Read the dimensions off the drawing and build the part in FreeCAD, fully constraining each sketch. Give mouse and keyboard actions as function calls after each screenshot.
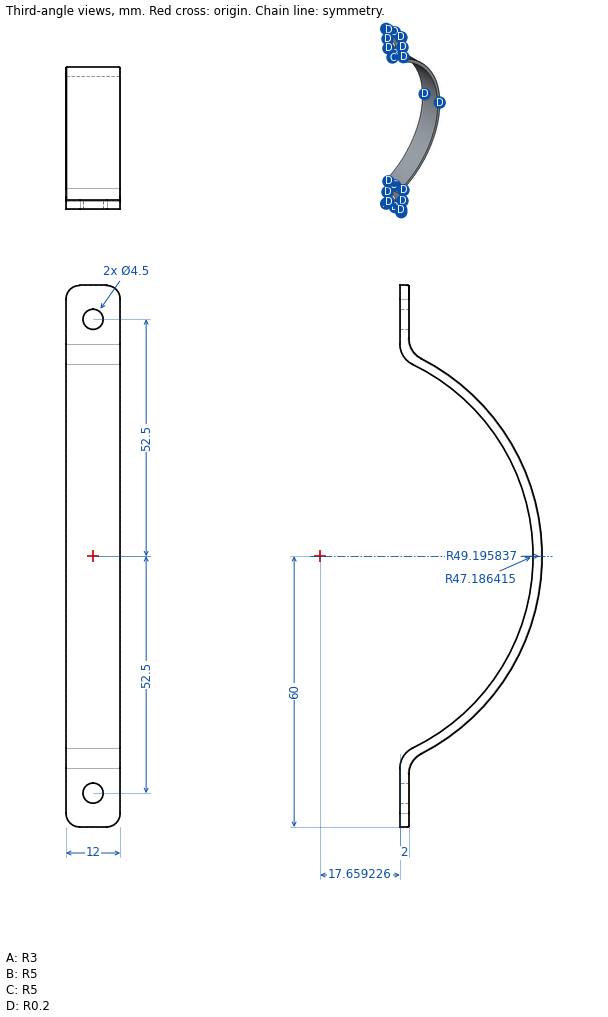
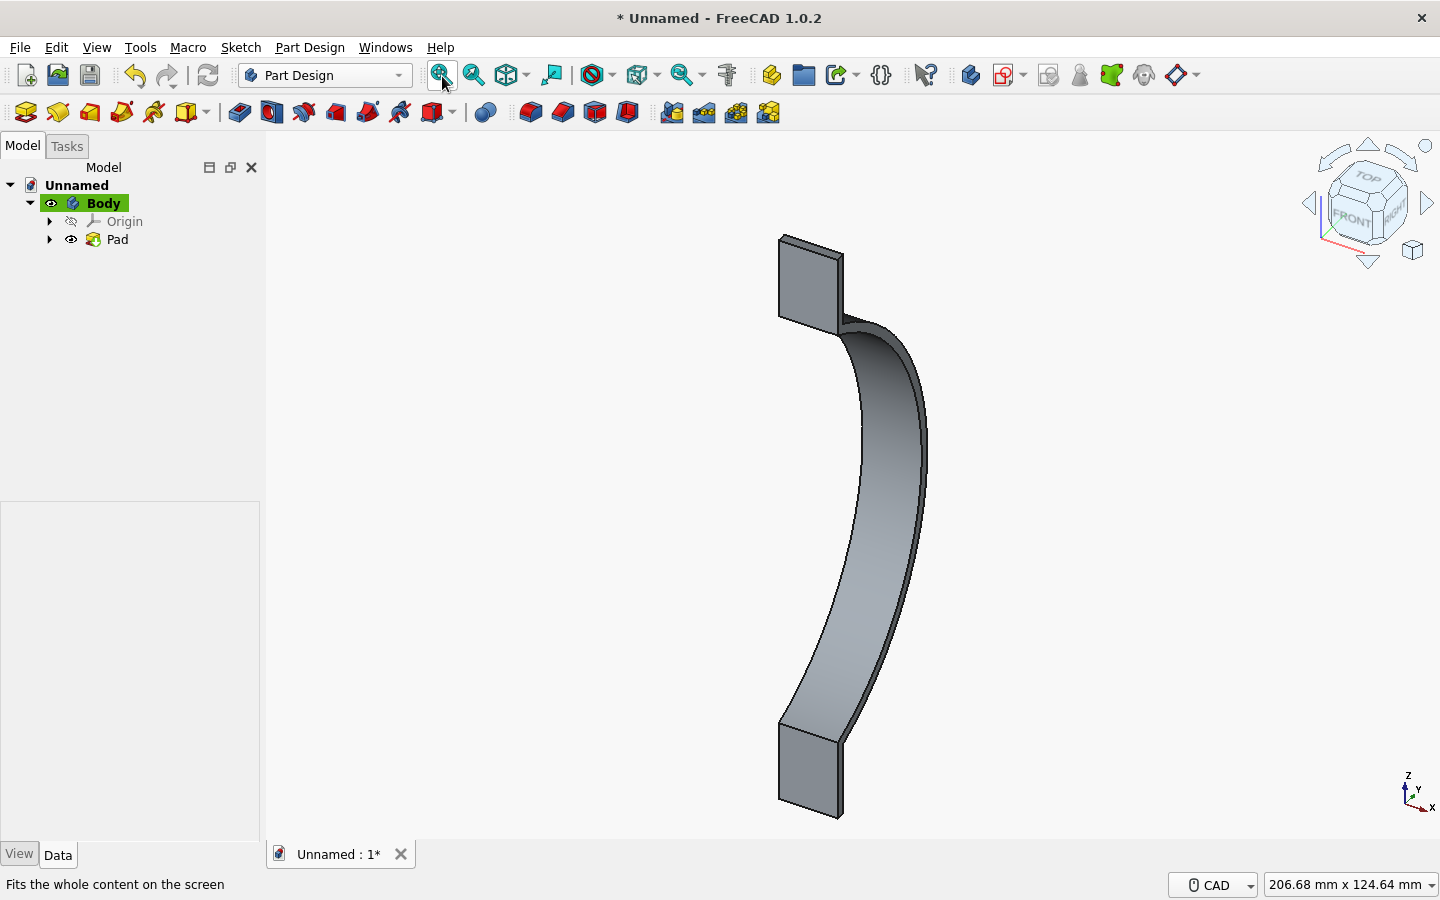
key(4)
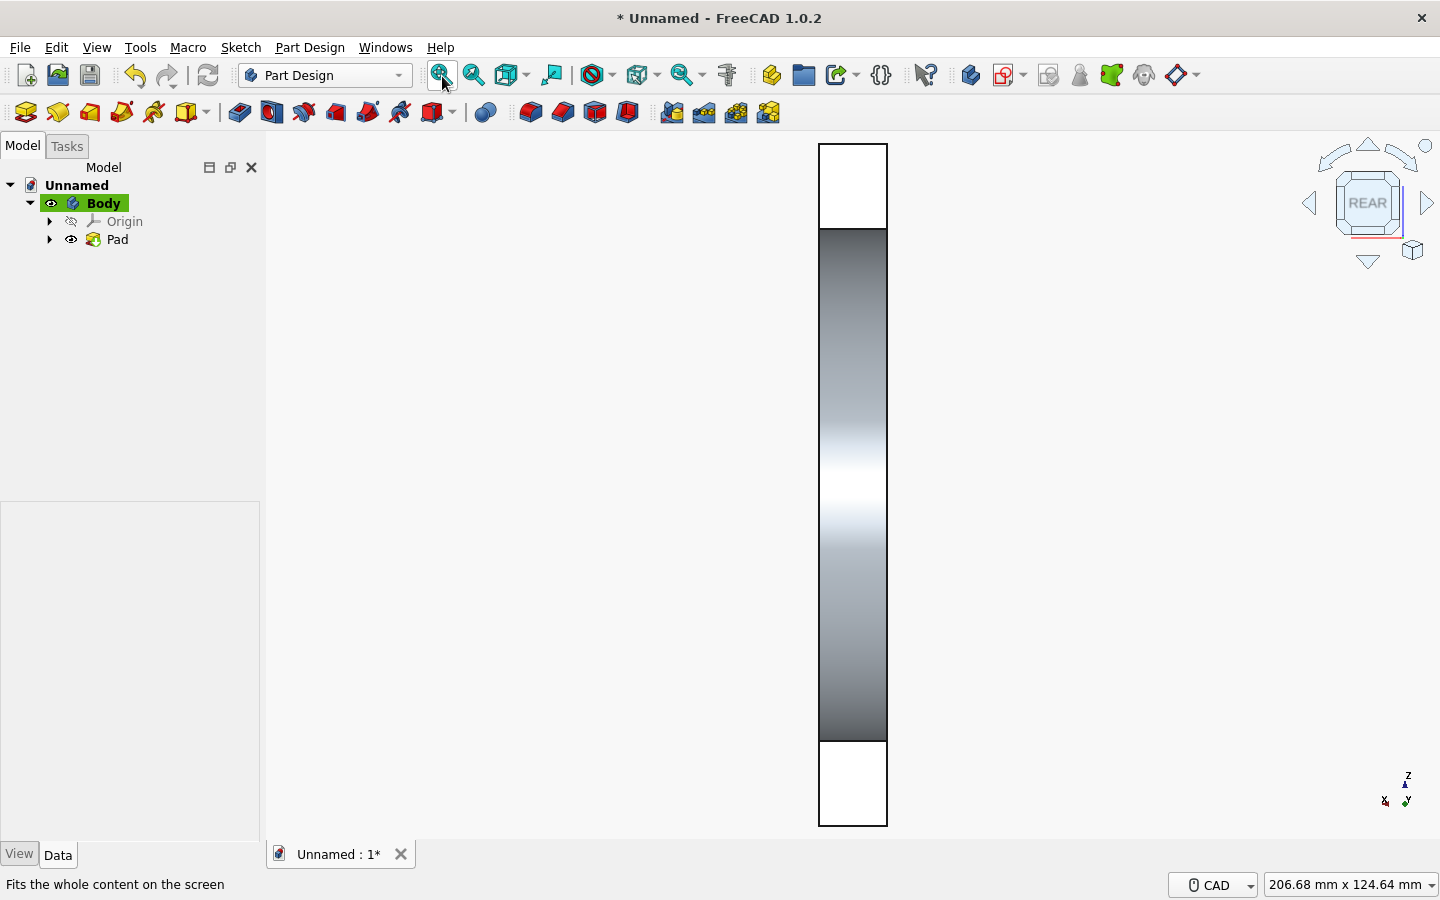
click(853, 186)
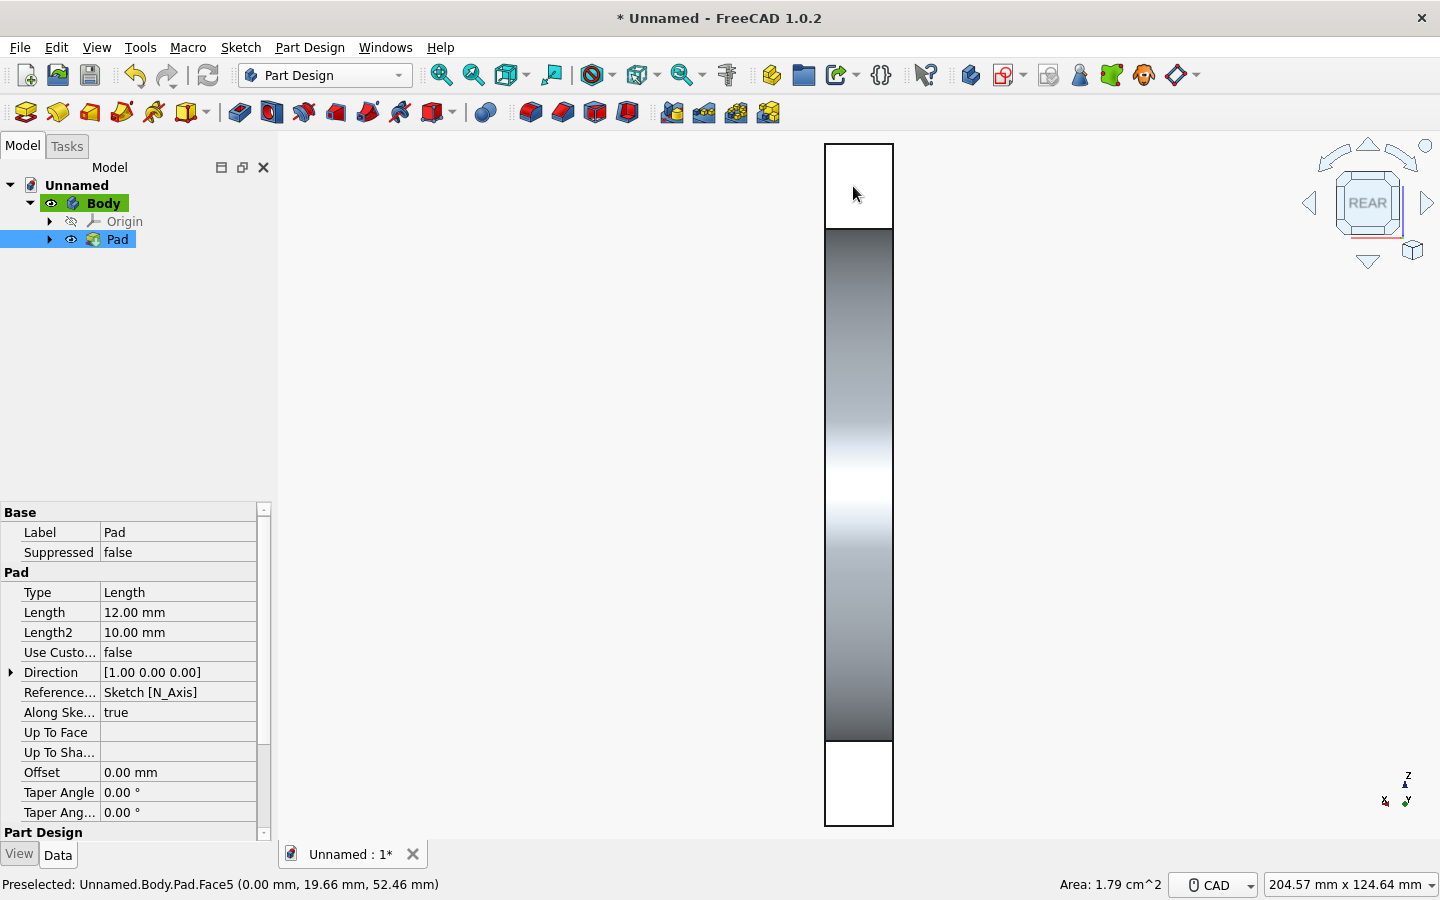
click(1004, 76)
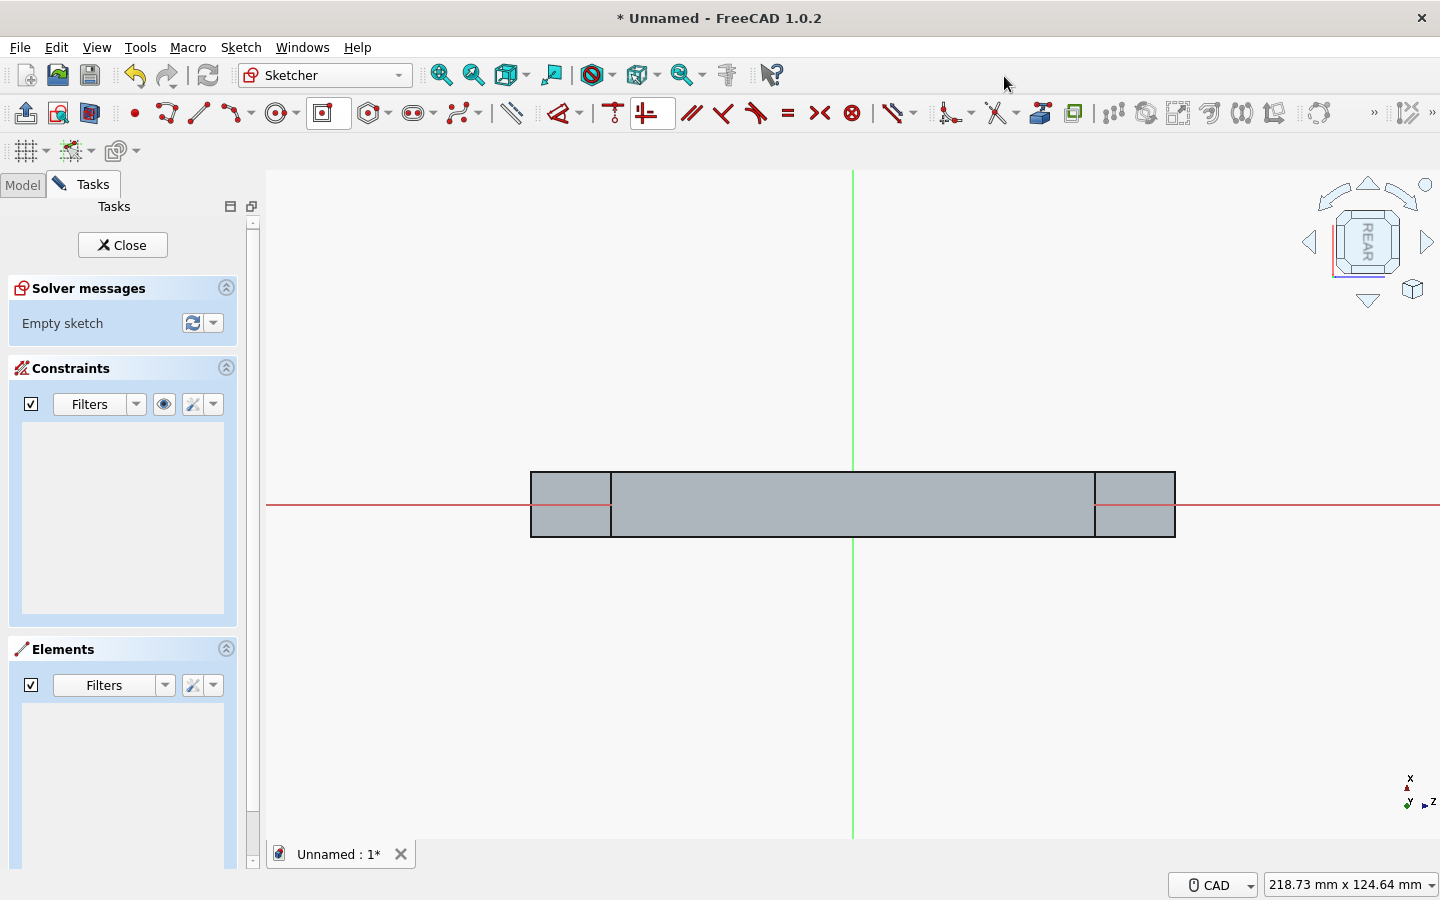
key(g)
key(c)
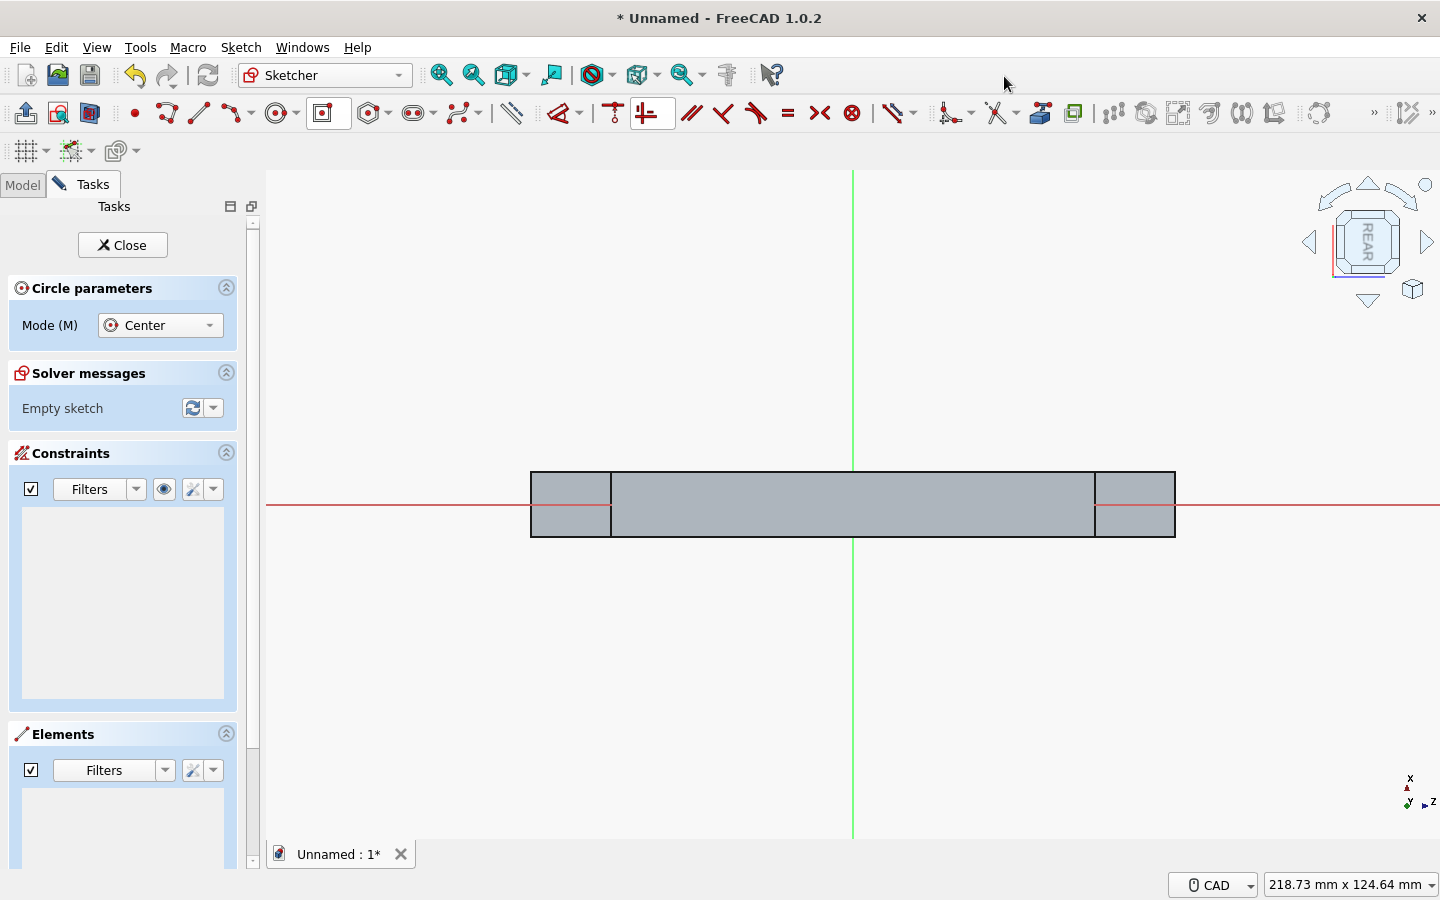
scroll(1135, 504, up, 4)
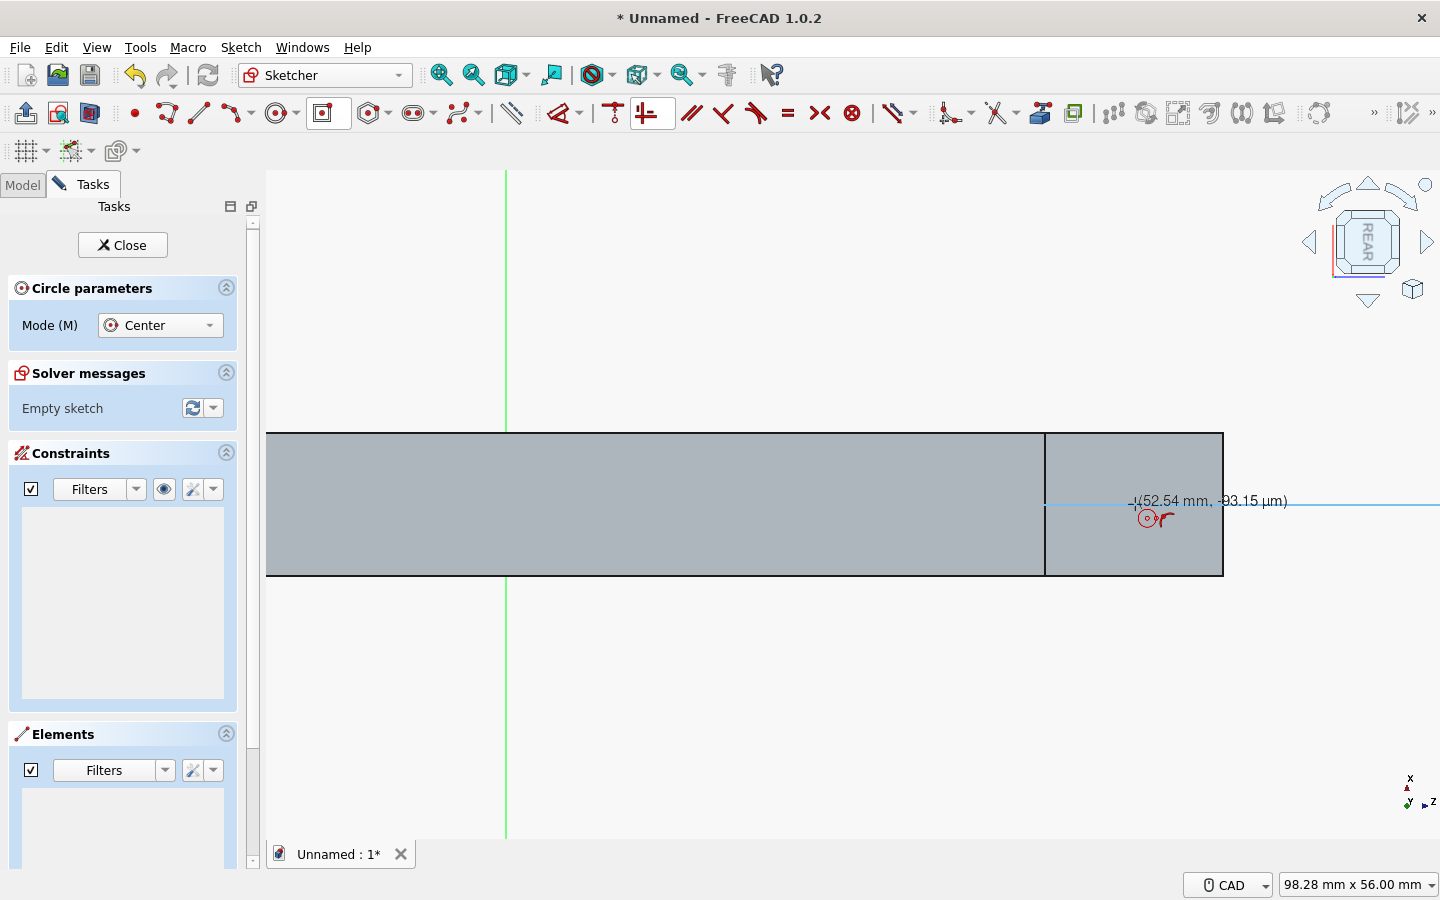
click(1134, 504)
move(1153, 485)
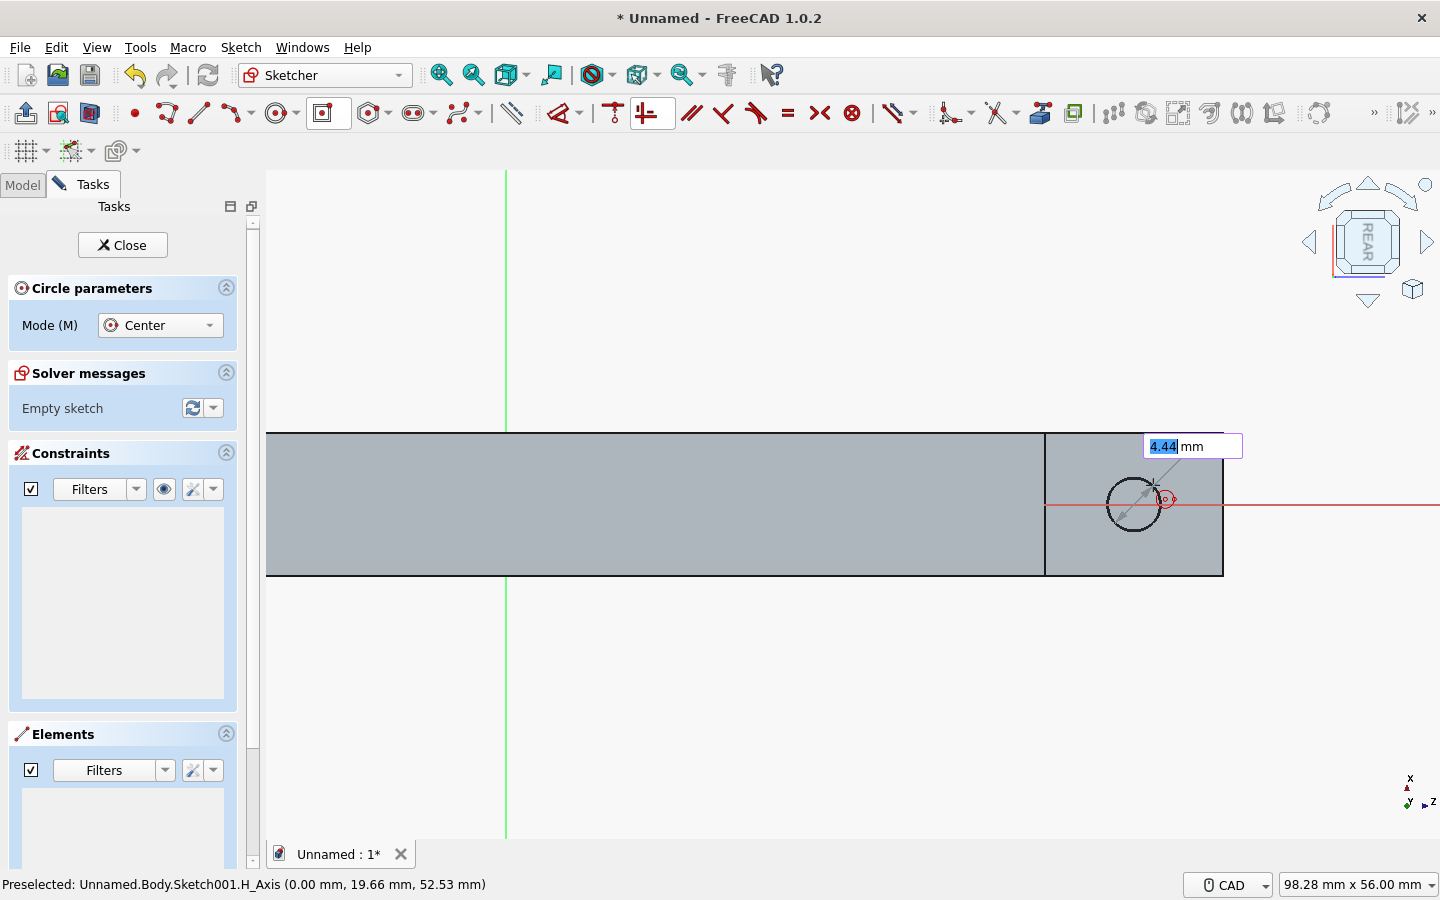
text(4.5)
key(Return)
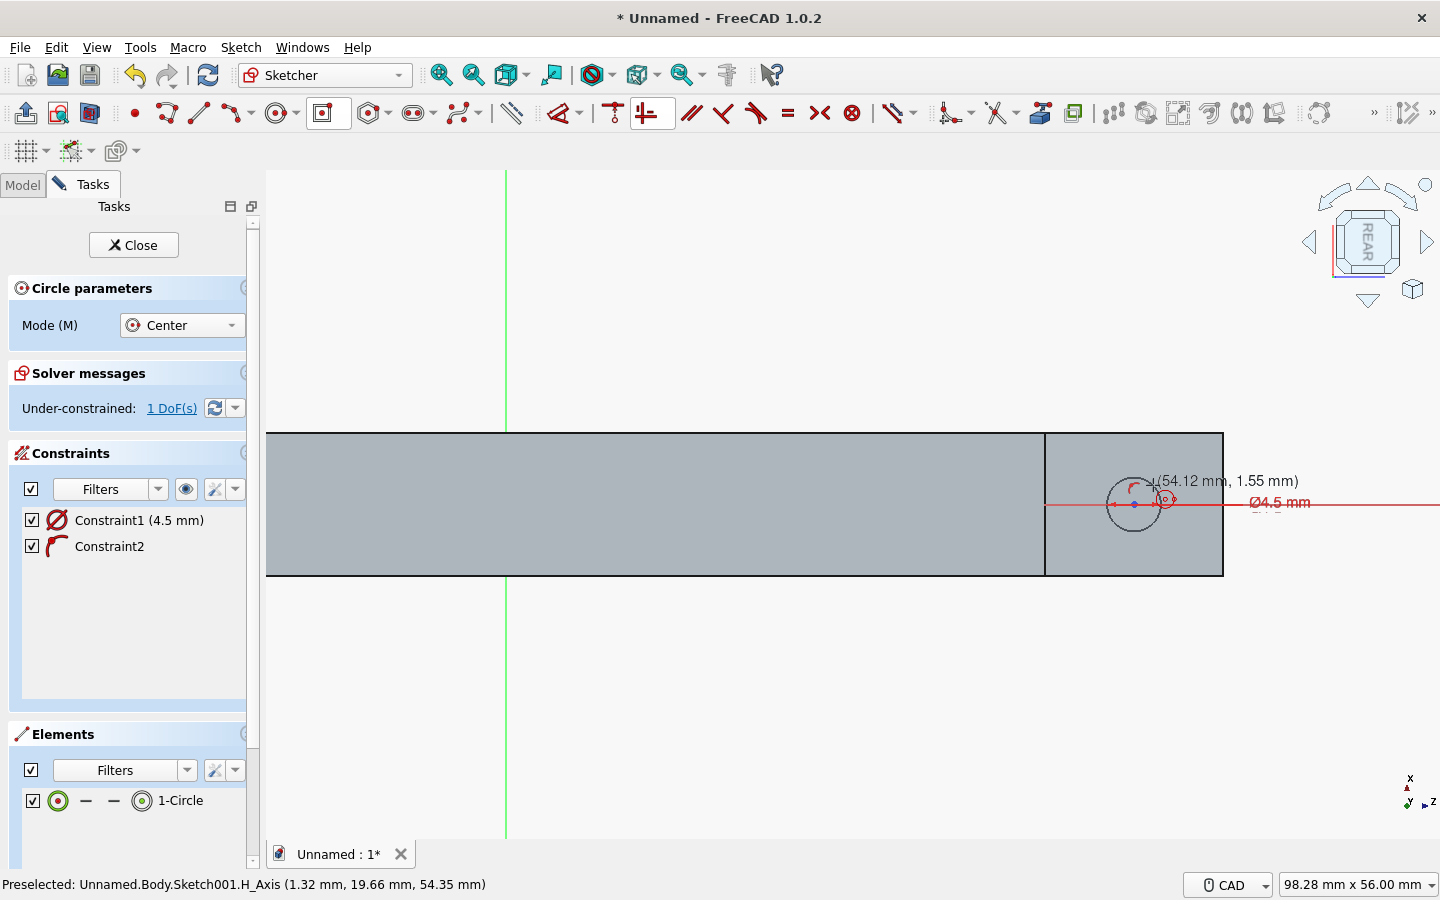
scroll(1123, 504, down, 3)